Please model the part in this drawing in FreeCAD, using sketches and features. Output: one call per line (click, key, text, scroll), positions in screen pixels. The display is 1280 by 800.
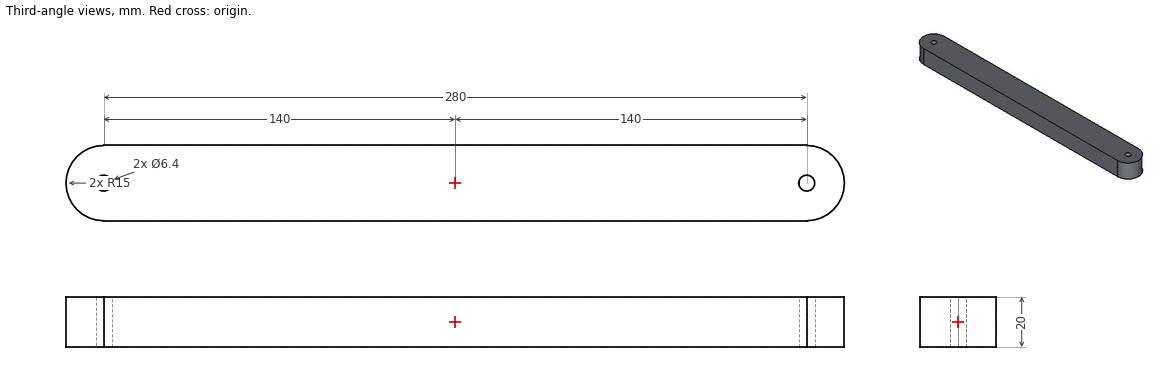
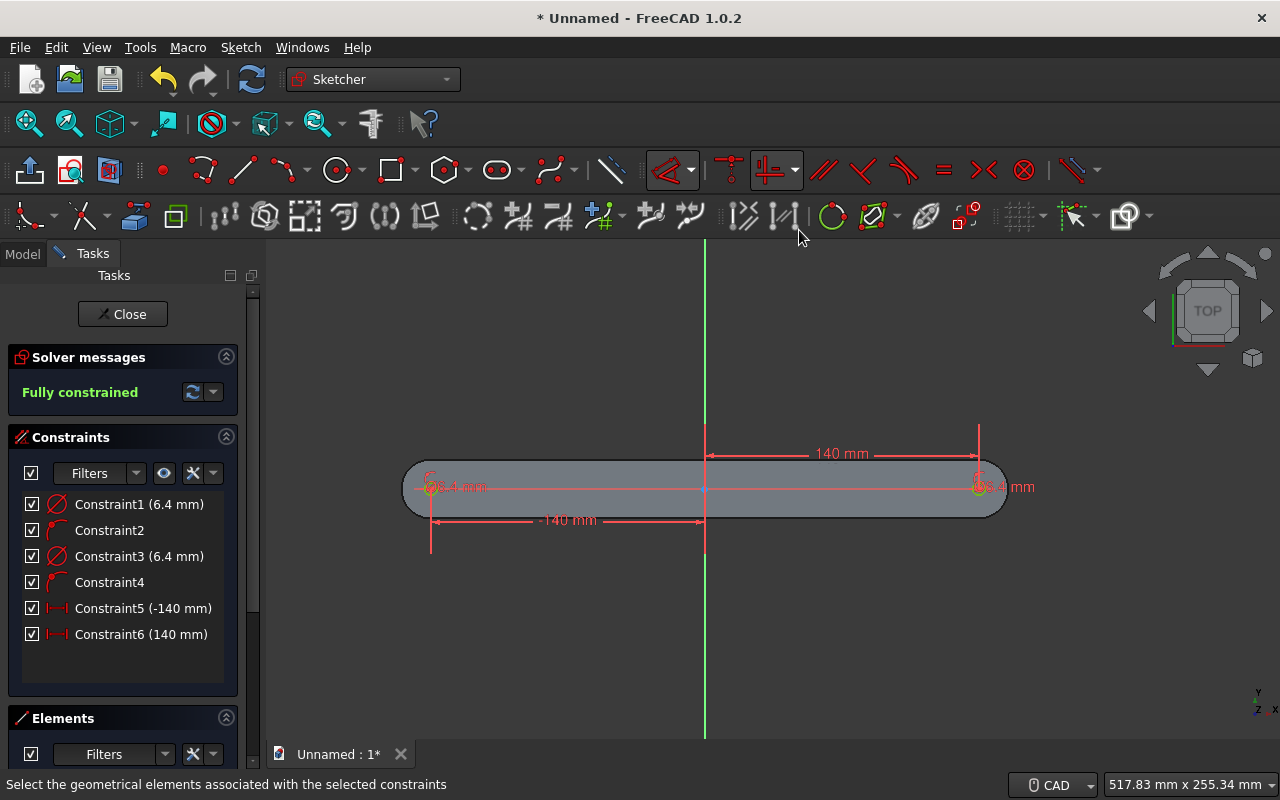
click(123, 314)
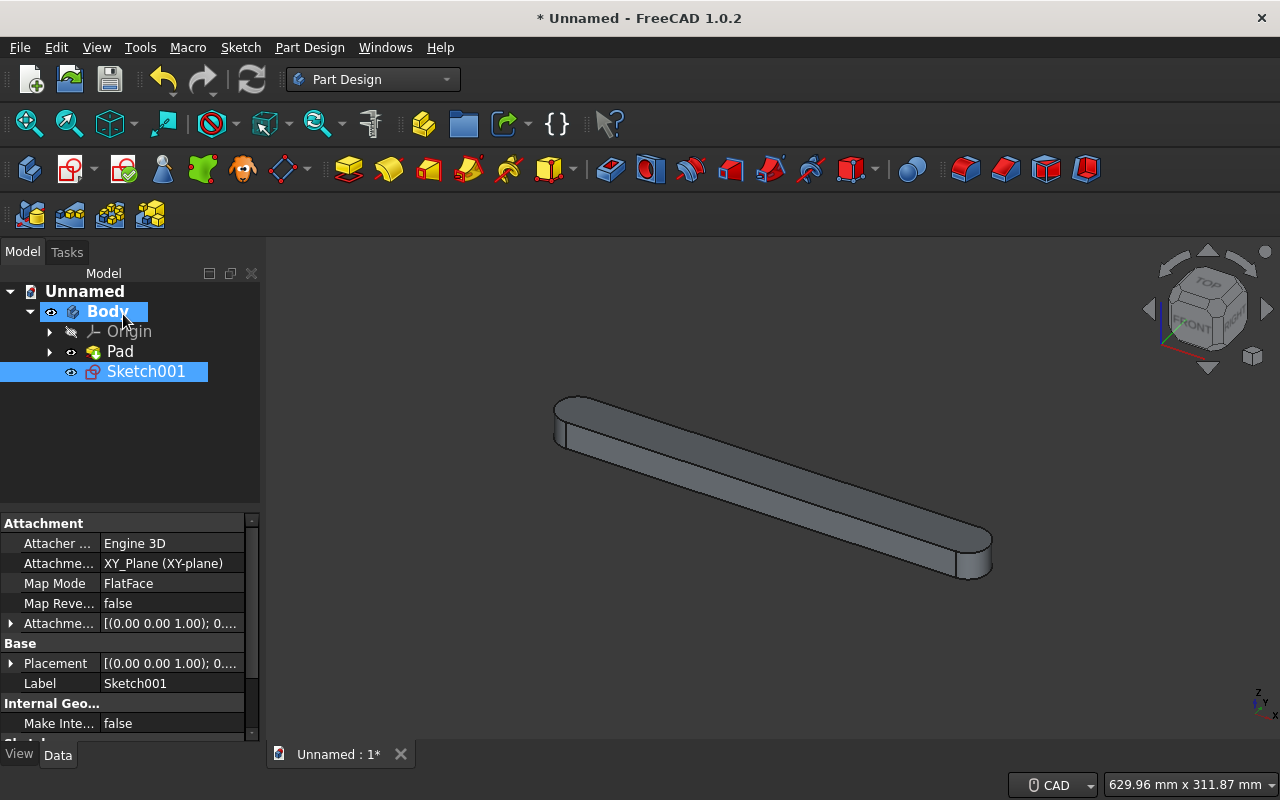
click(612, 170)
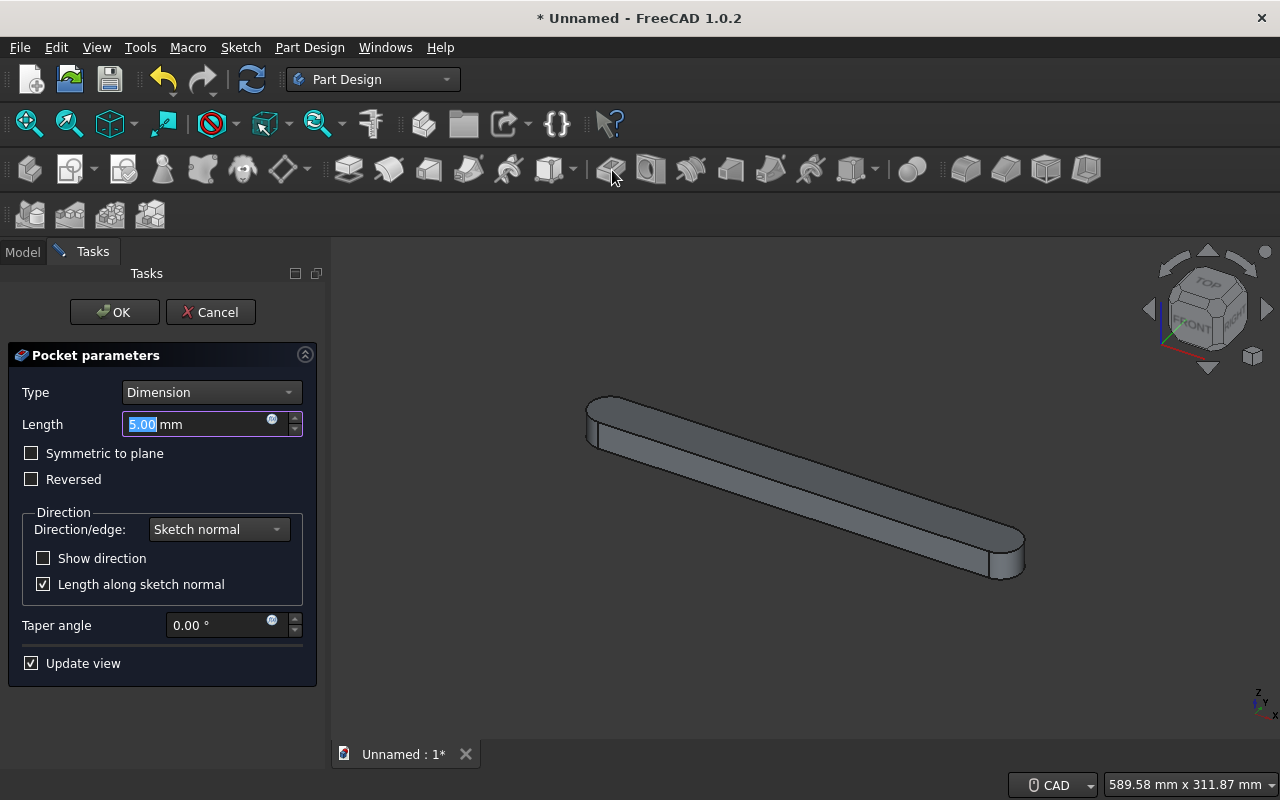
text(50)
key(Tab)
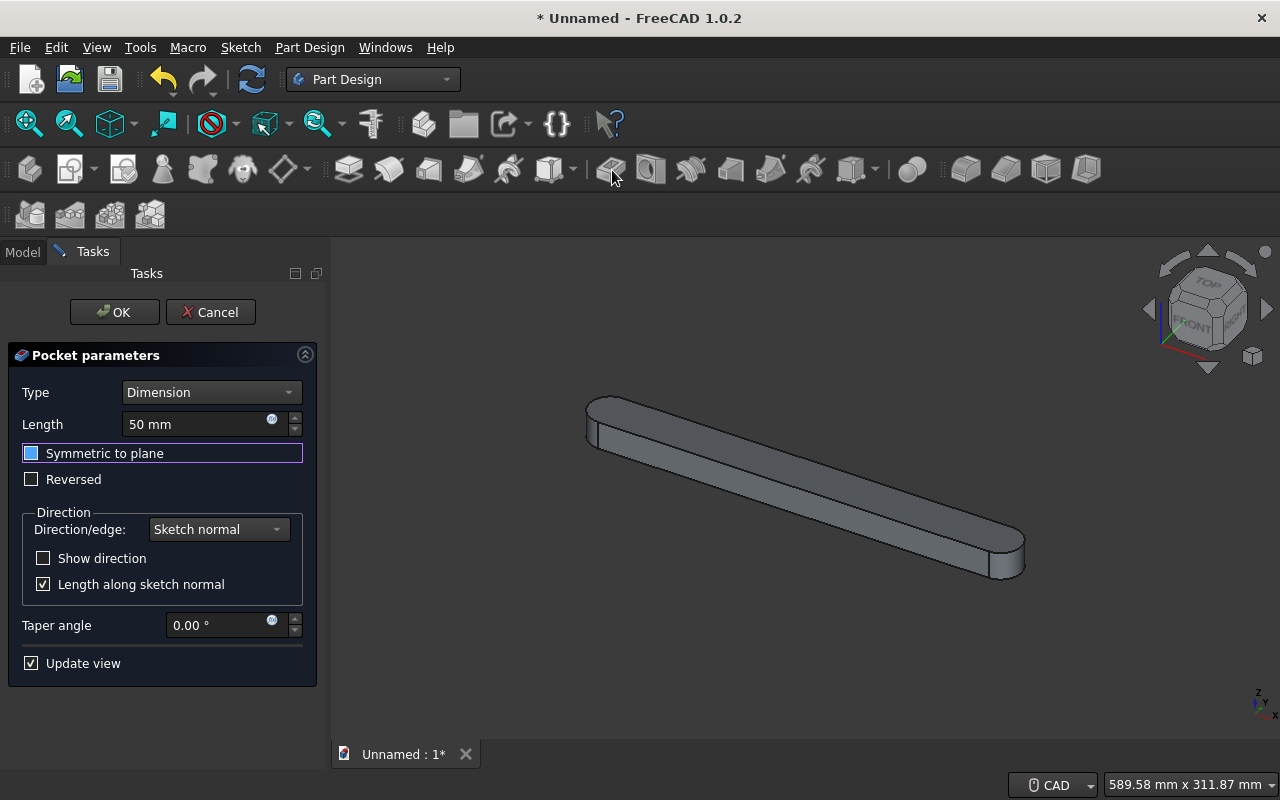
click(30, 453)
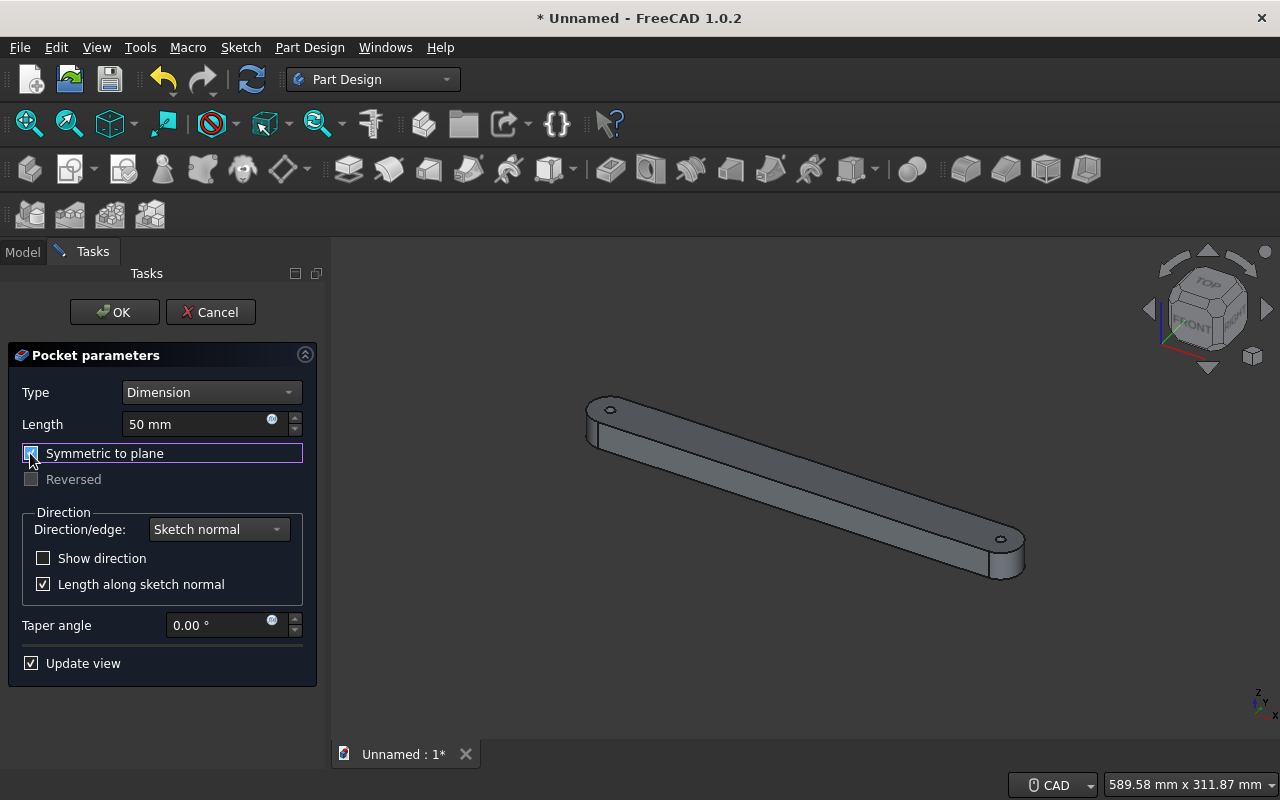
click(115, 312)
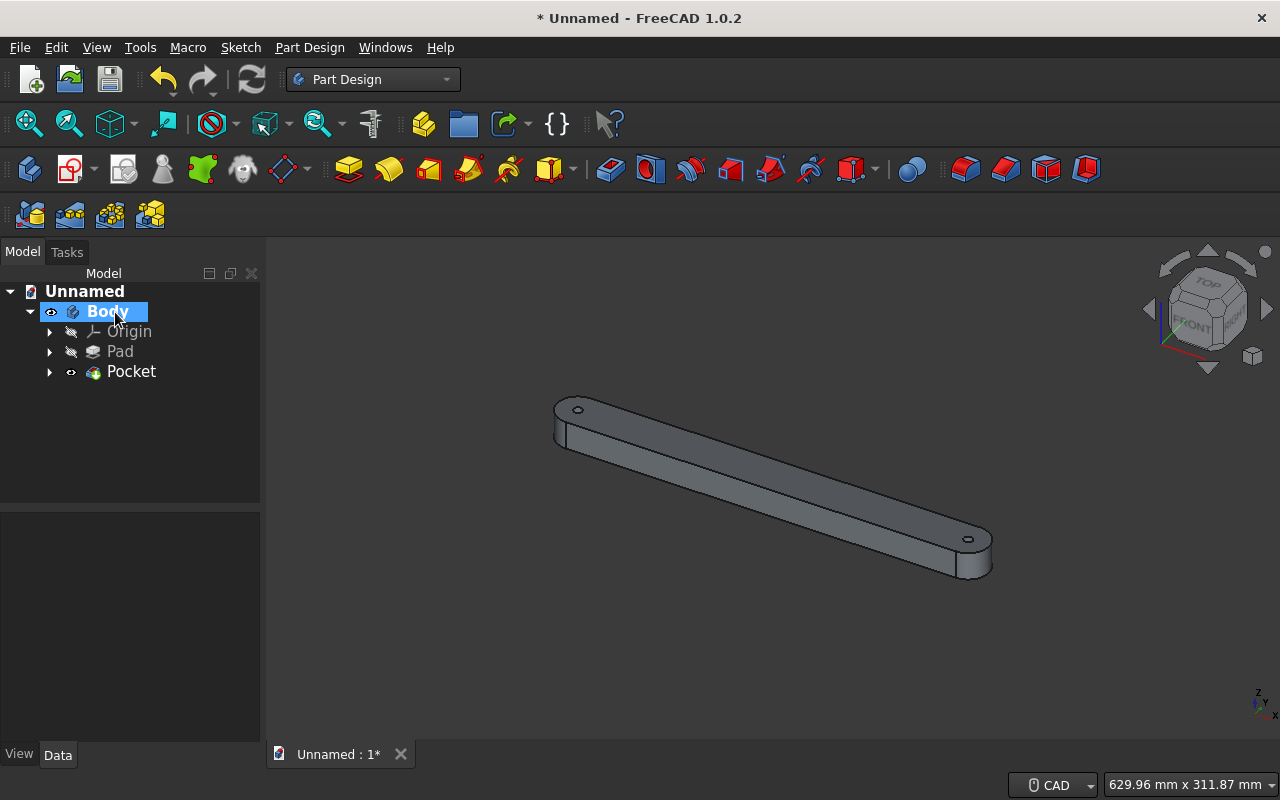
key(0)